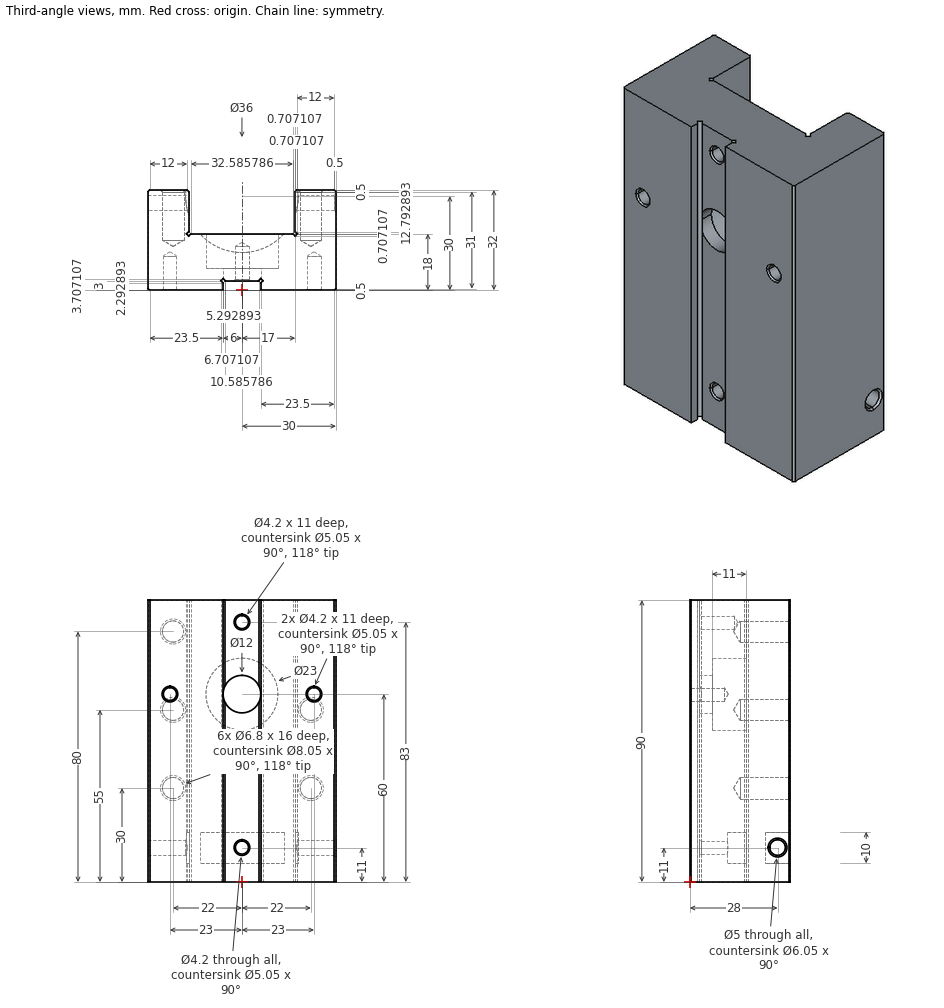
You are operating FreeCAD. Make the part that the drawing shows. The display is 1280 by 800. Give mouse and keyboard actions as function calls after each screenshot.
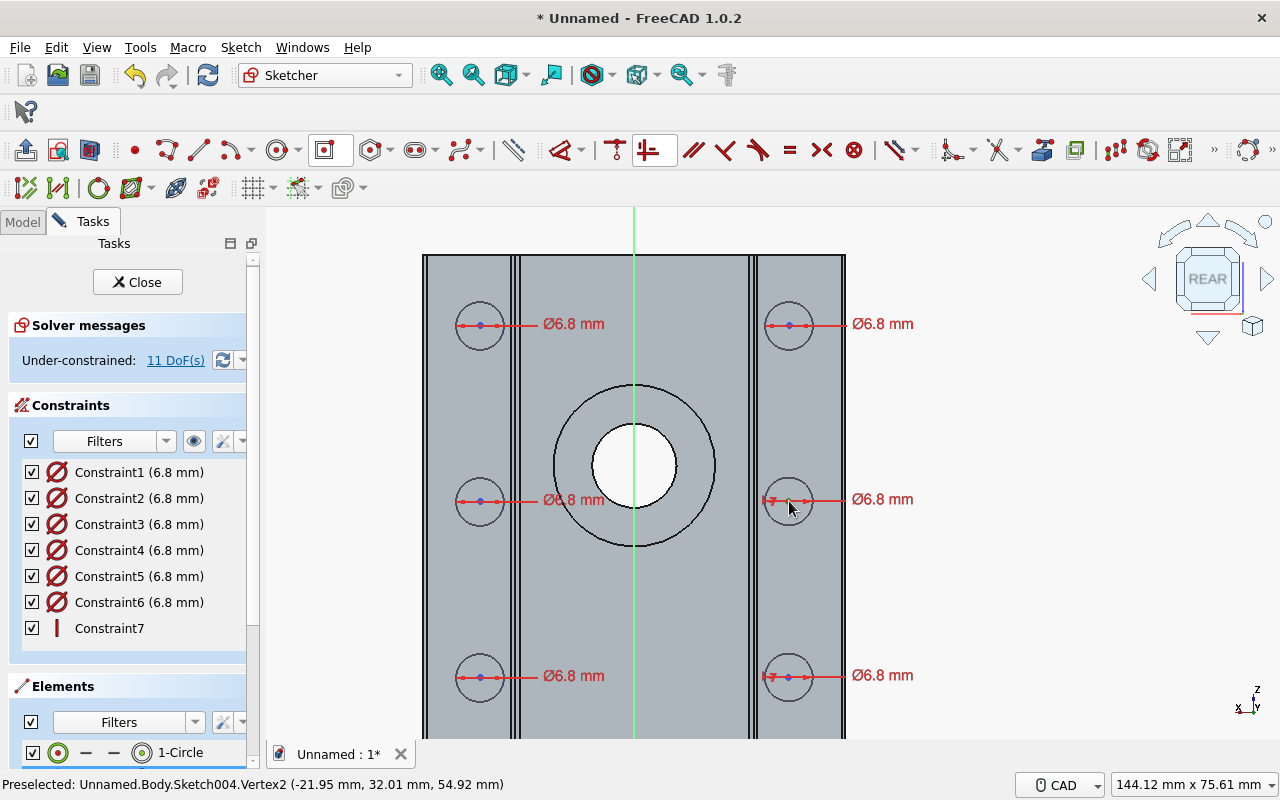
click(789, 326)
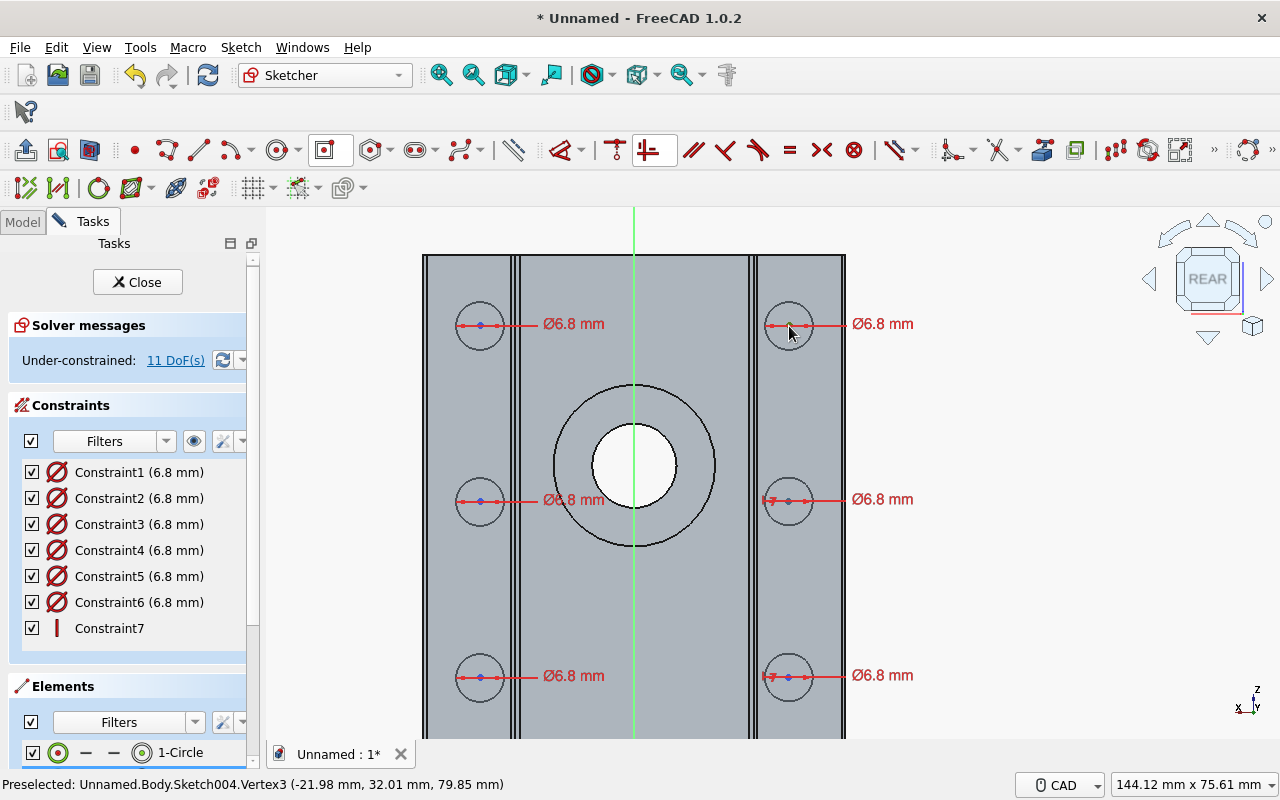
key(v)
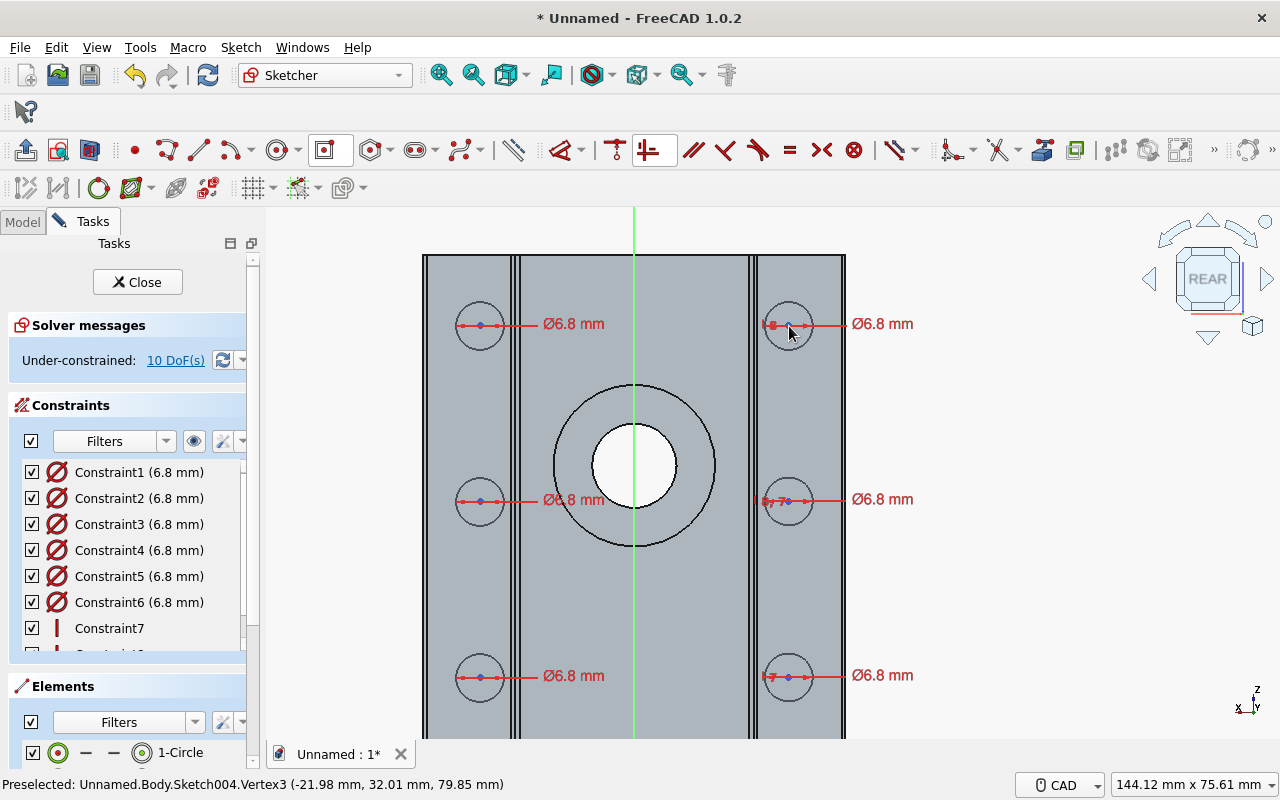
click(789, 677)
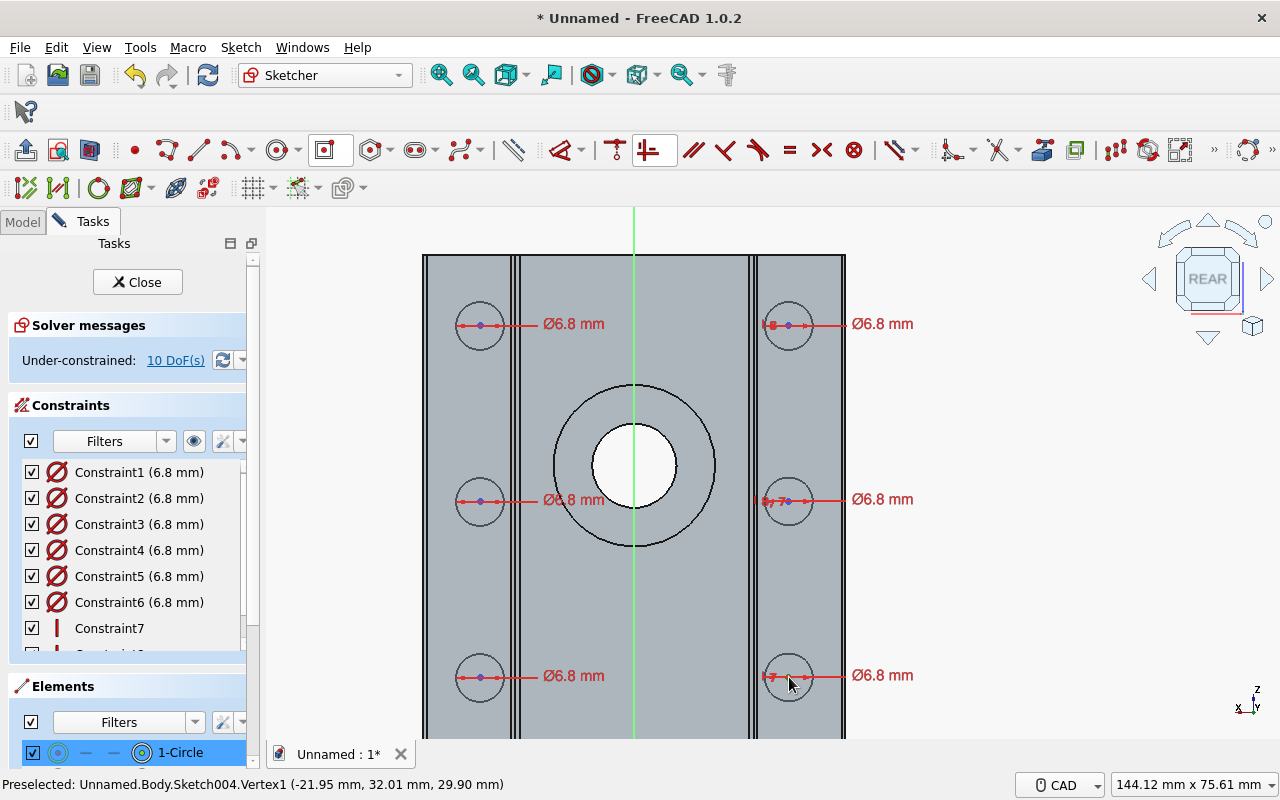
click(480, 678)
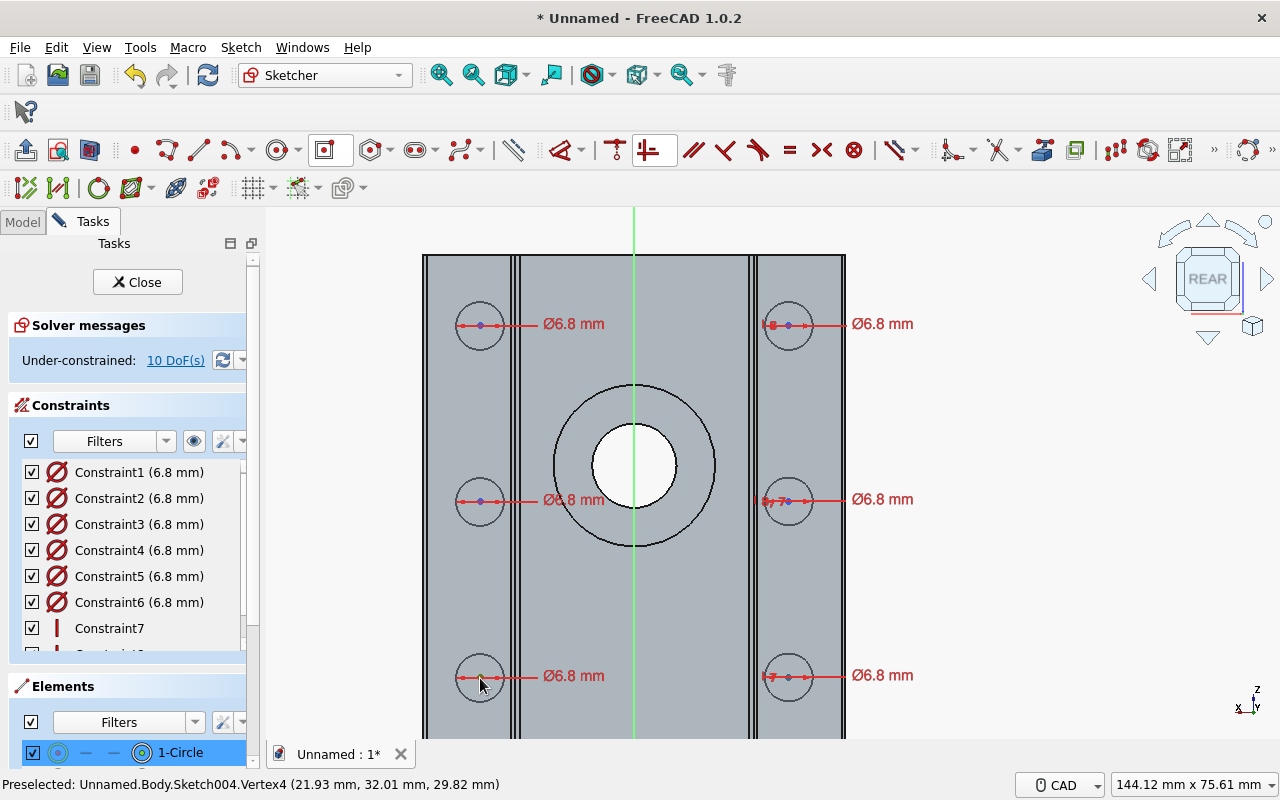
click(672, 150)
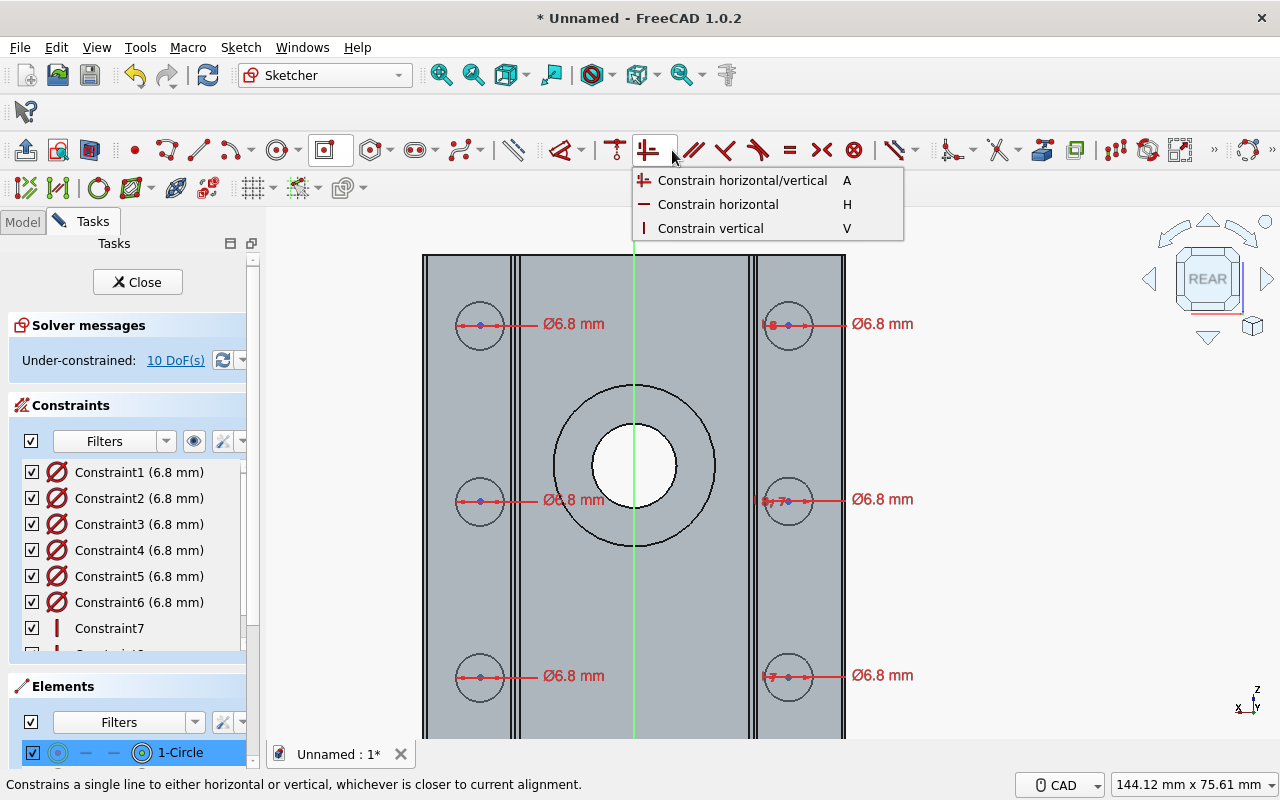
click(768, 204)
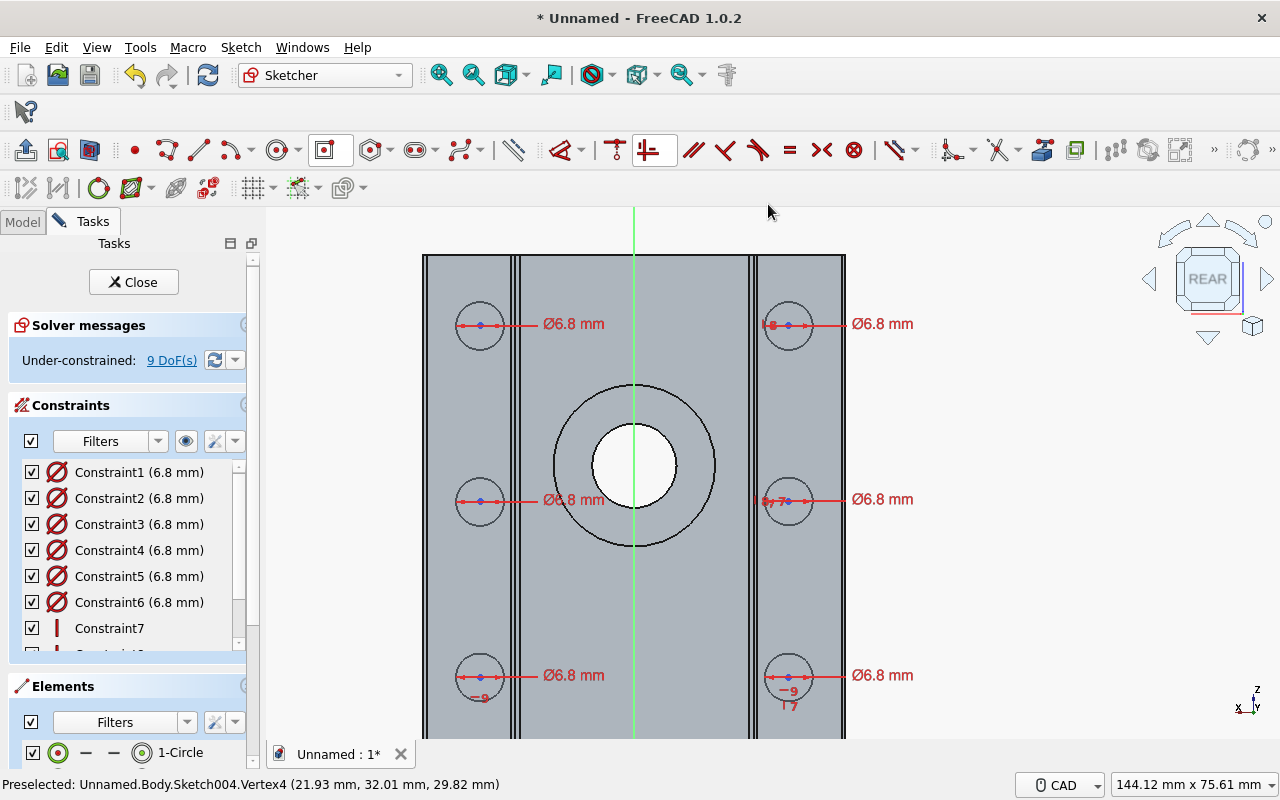
click(480, 677)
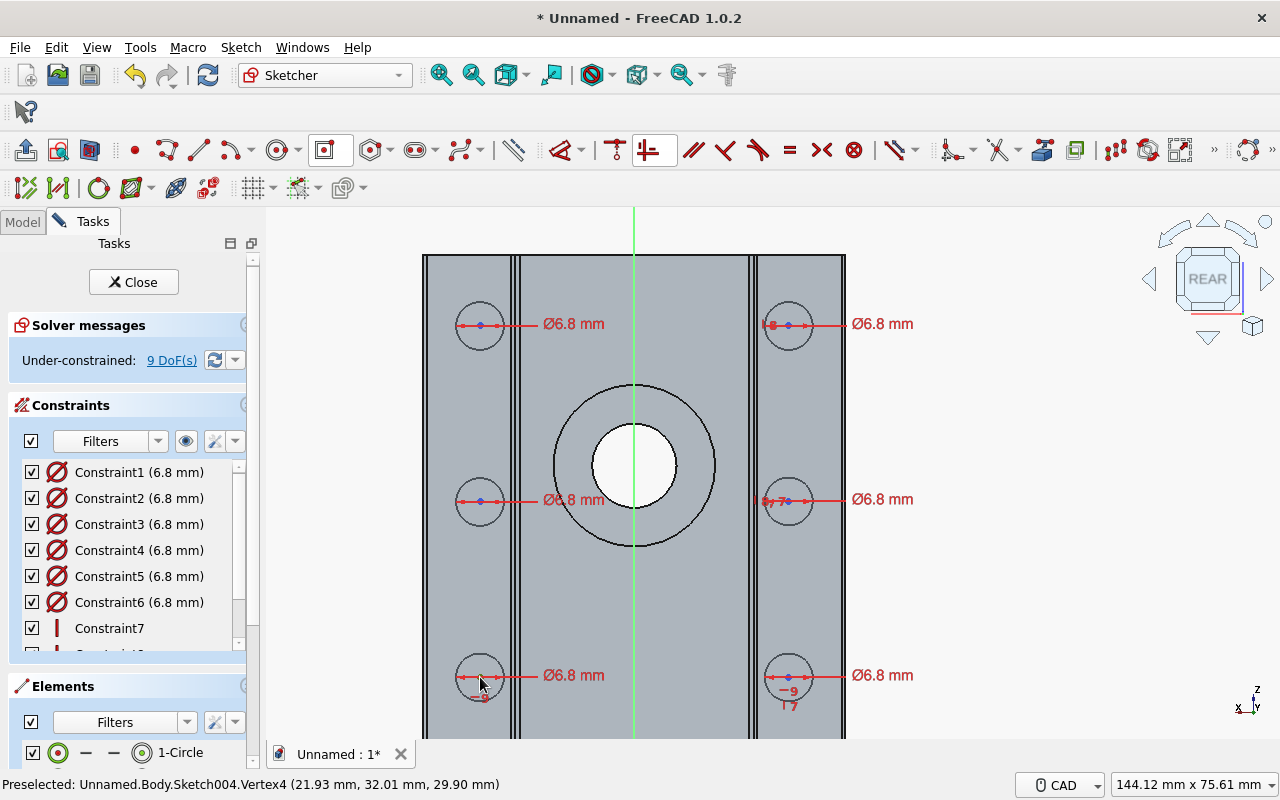
click(480, 502)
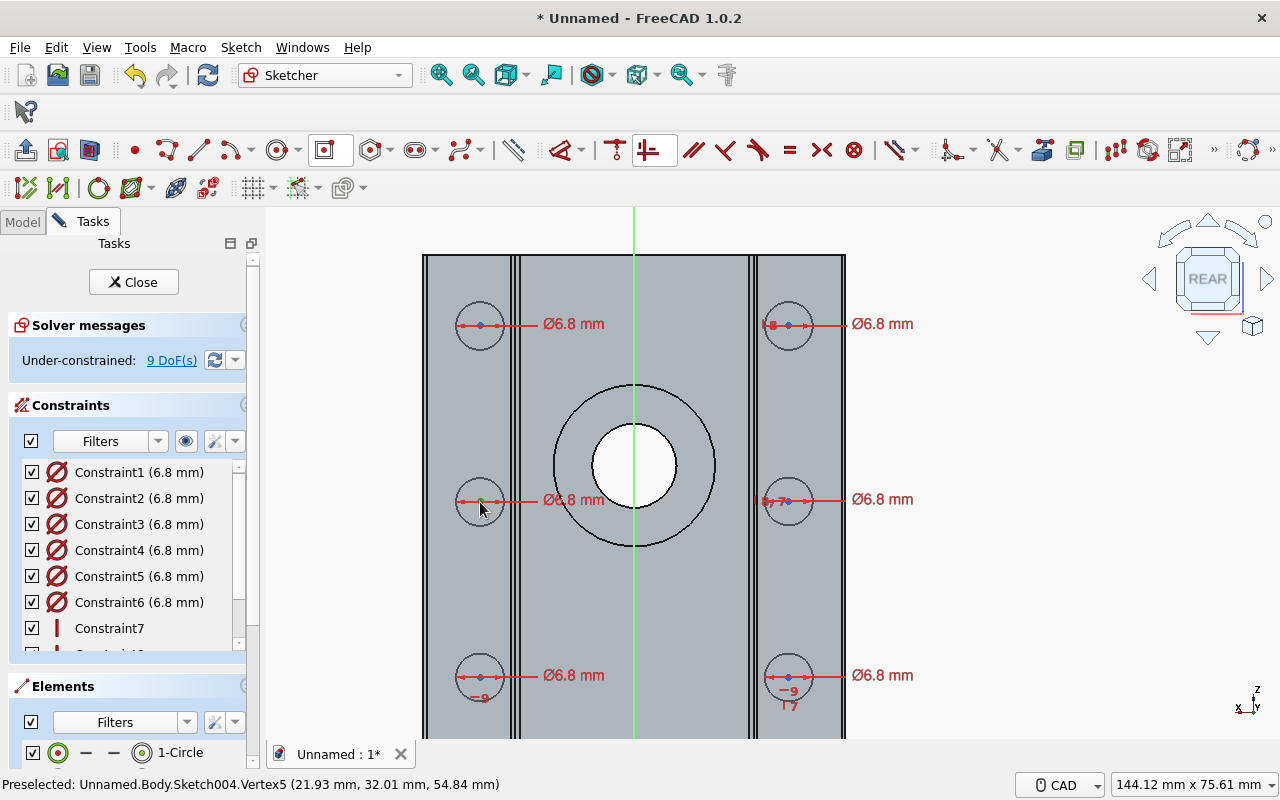
key(v)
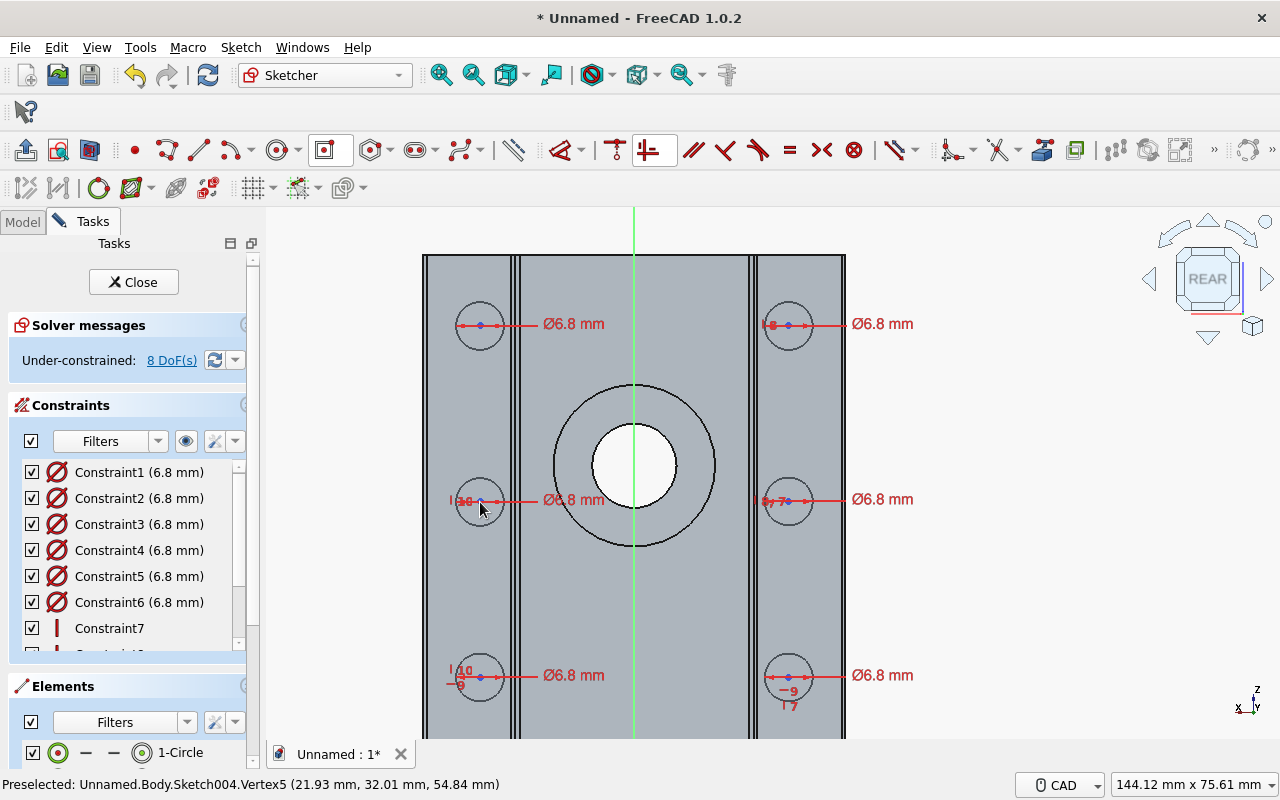
click(789, 501)